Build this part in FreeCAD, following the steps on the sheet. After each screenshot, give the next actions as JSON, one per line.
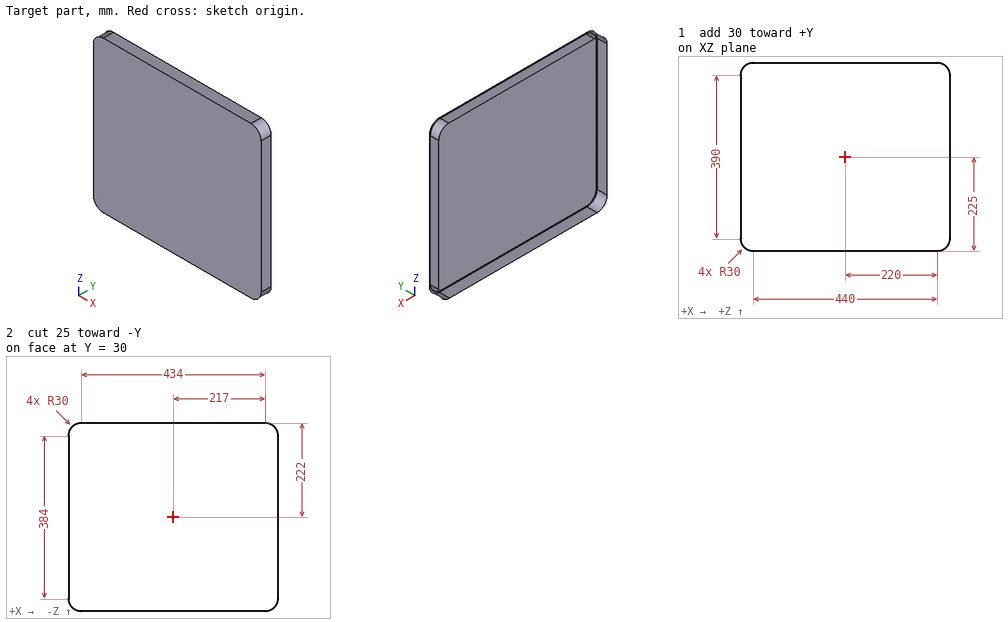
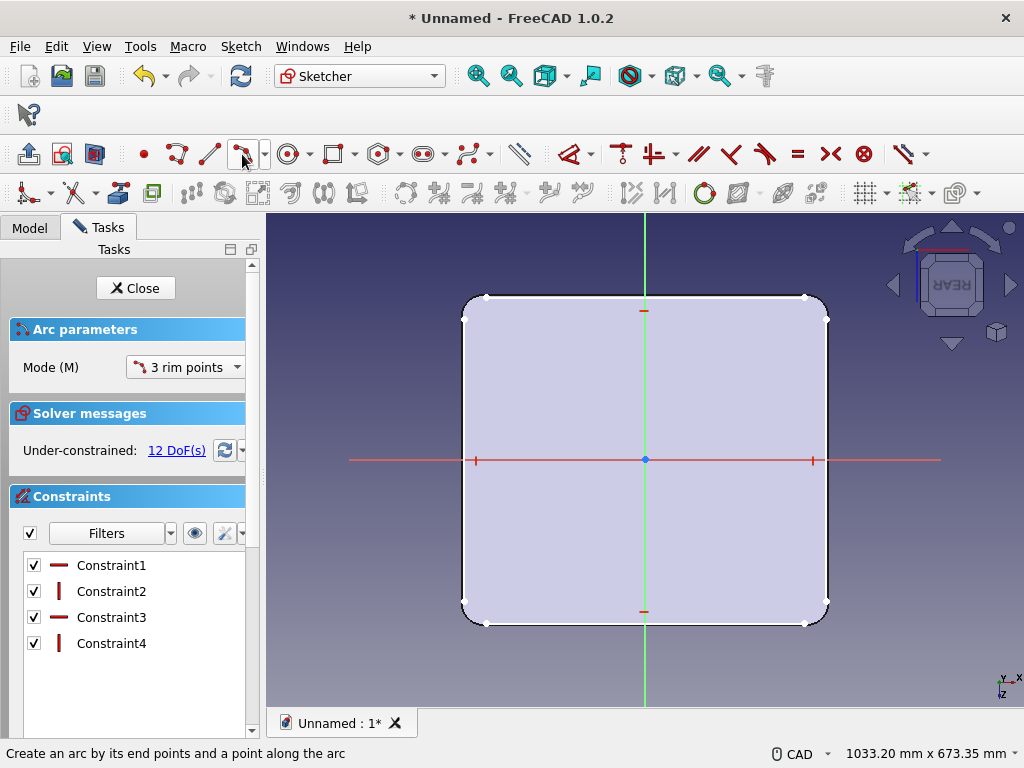
{"action": "left_click", "coordinate": [486, 298]}
{"action": "left_click", "coordinate": [464, 320]}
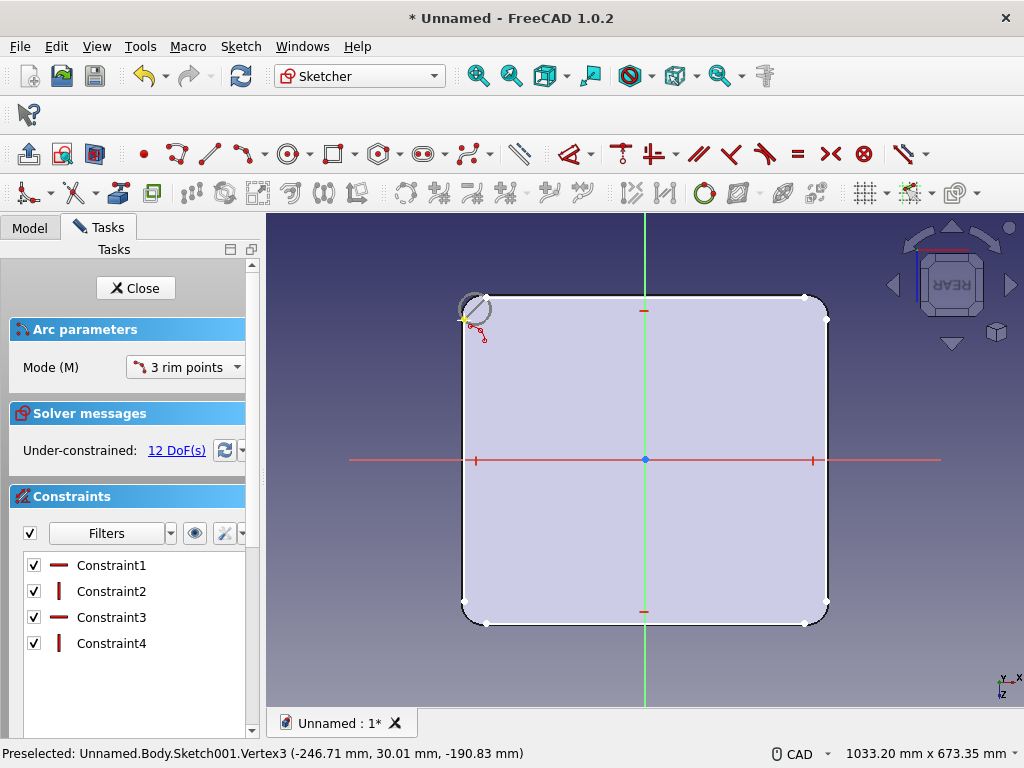
{"action": "scroll", "coordinate": [470, 304], "scroll_direction": "up", "scroll_amount": 5}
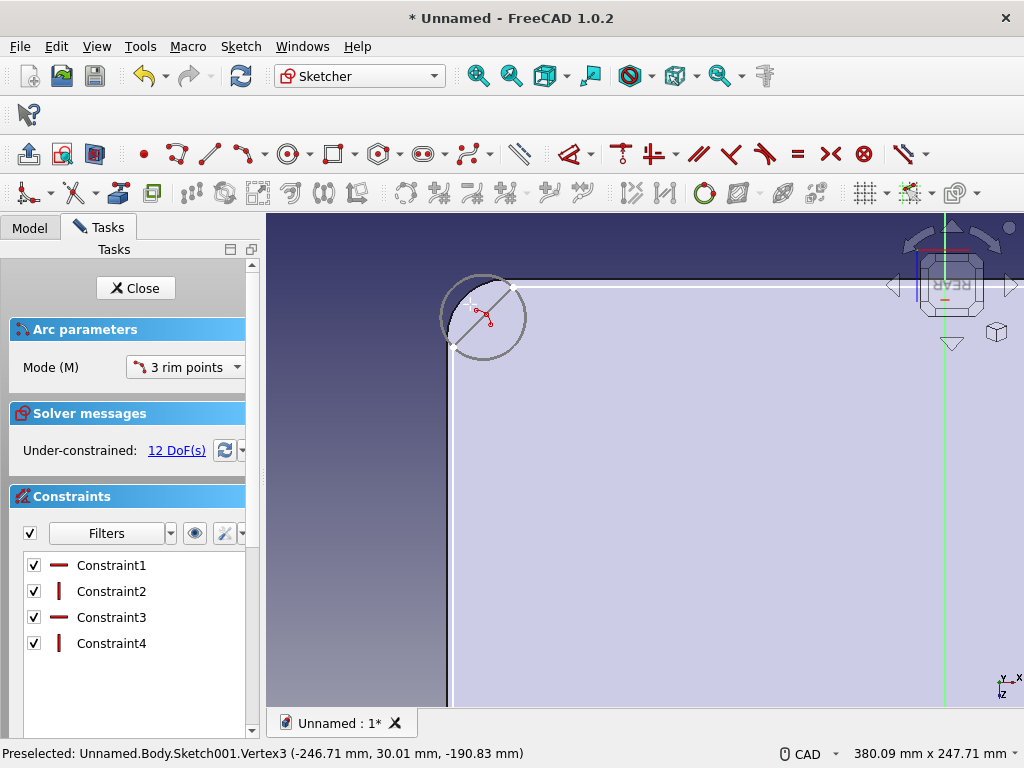
{"action": "left_click", "coordinate": [470, 303]}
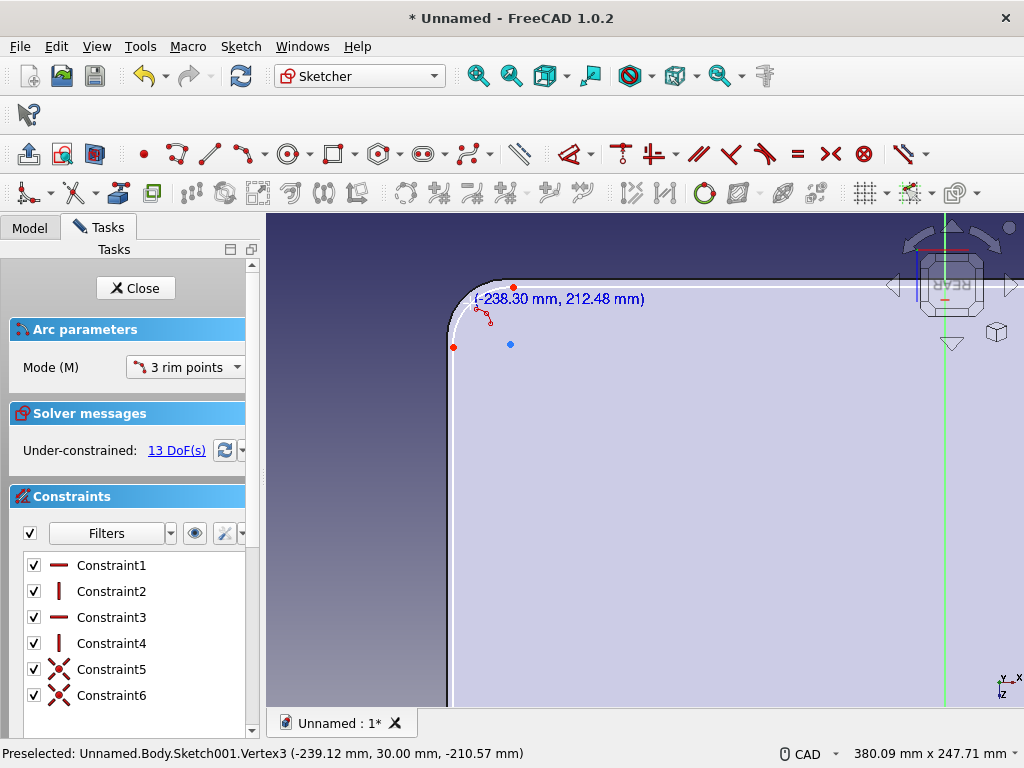
{"action": "scroll", "coordinate": [362, 304], "scroll_direction": "down", "scroll_amount": 5}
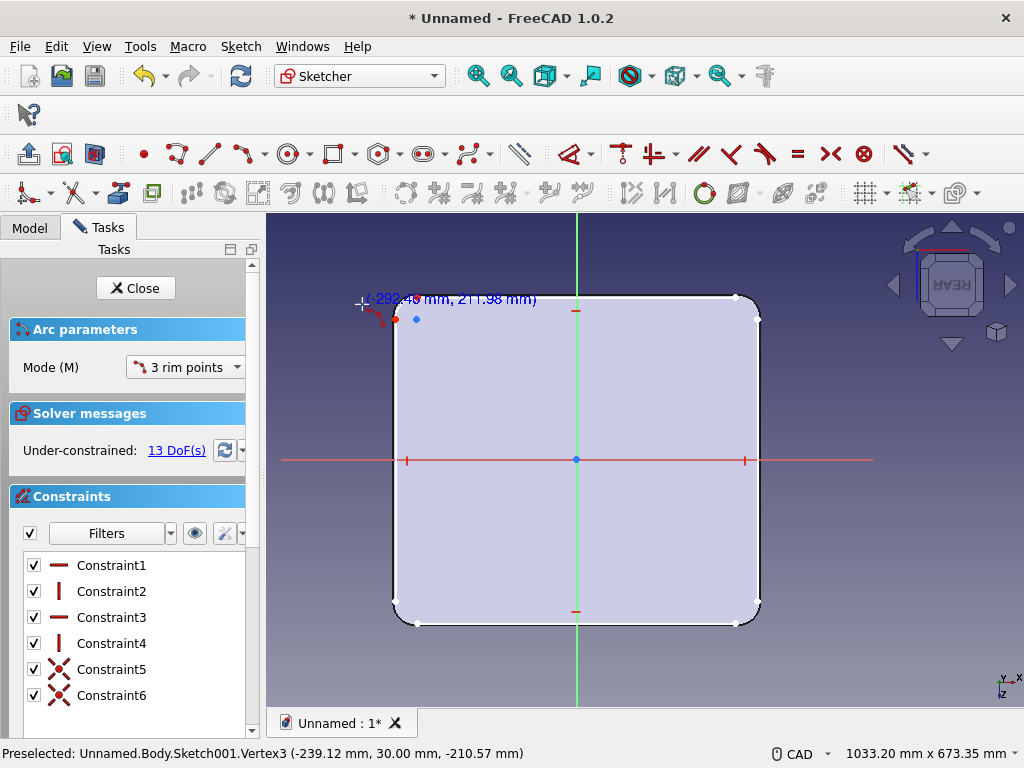
{"action": "left_click", "coordinate": [396, 602]}
{"action": "left_click", "coordinate": [418, 624]}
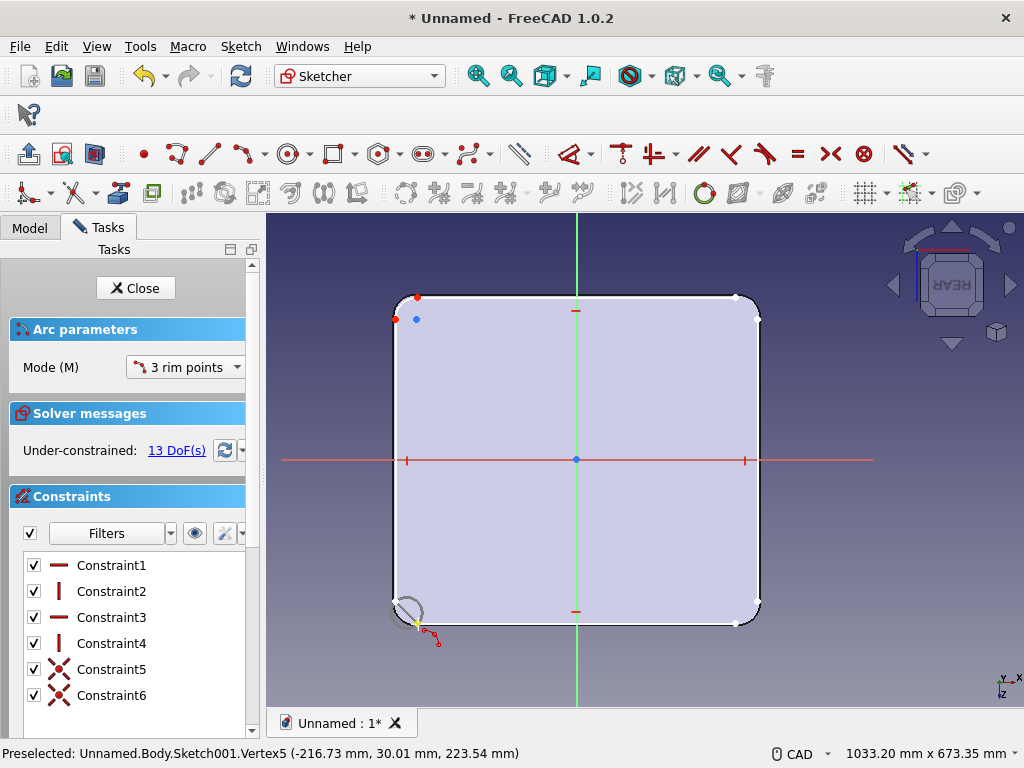
{"action": "scroll", "coordinate": [402, 616], "scroll_direction": "up", "scroll_amount": 5}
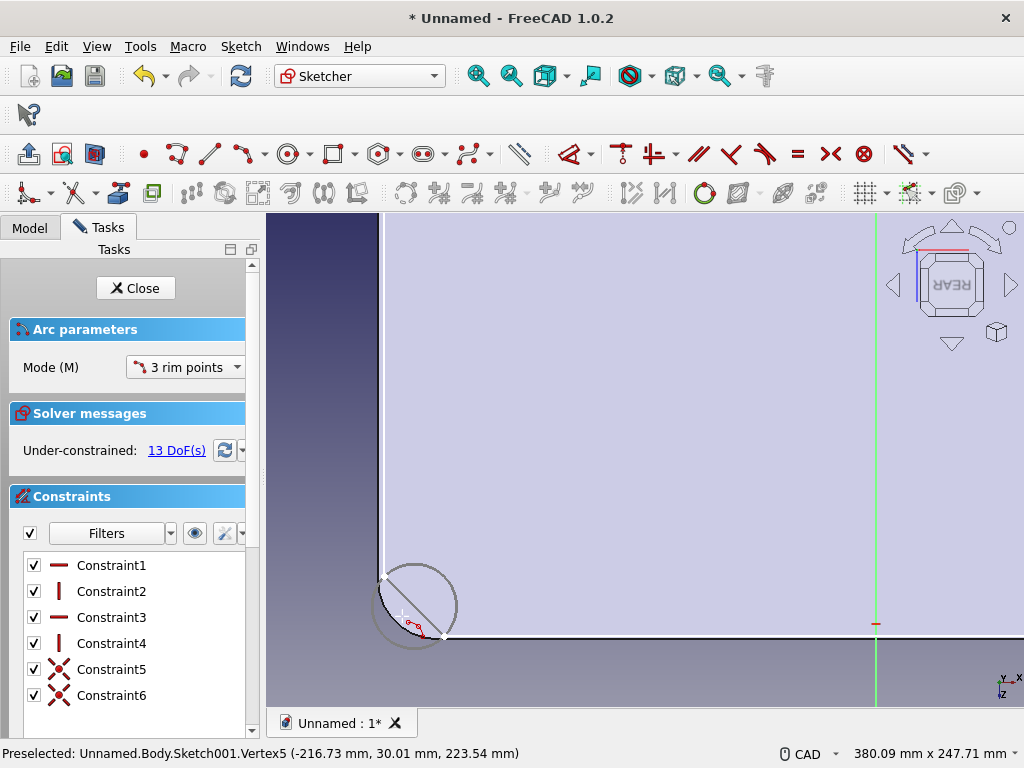
{"action": "left_click", "coordinate": [401, 616]}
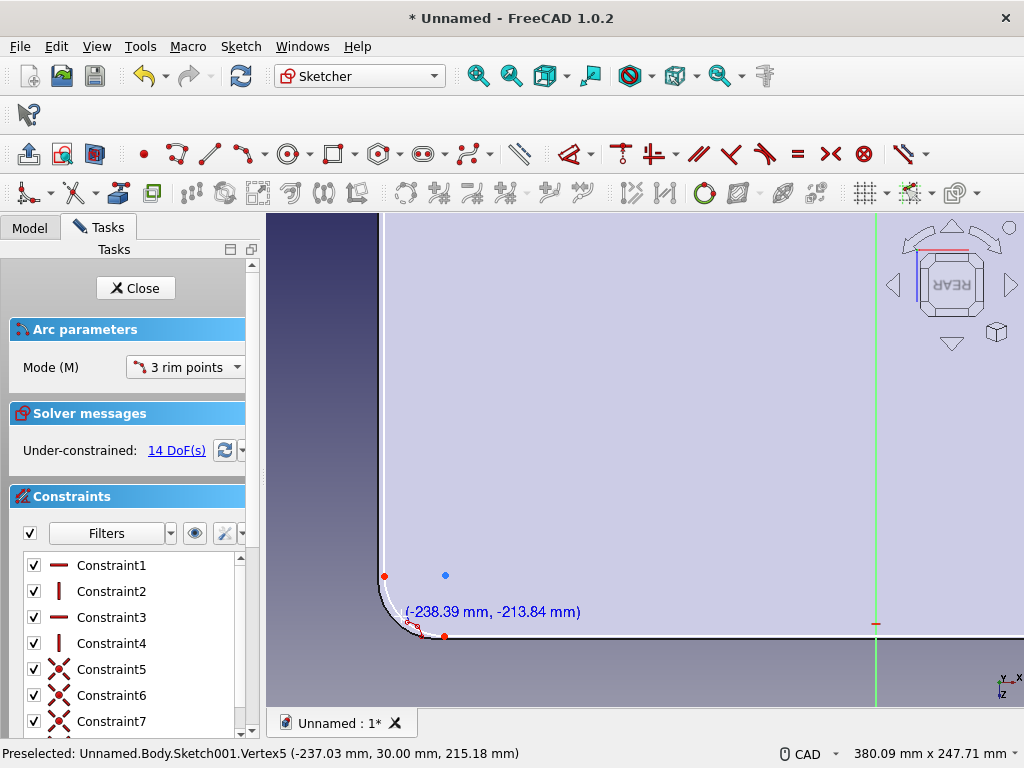
{"action": "scroll", "coordinate": [402, 617], "scroll_direction": "down", "scroll_amount": 5}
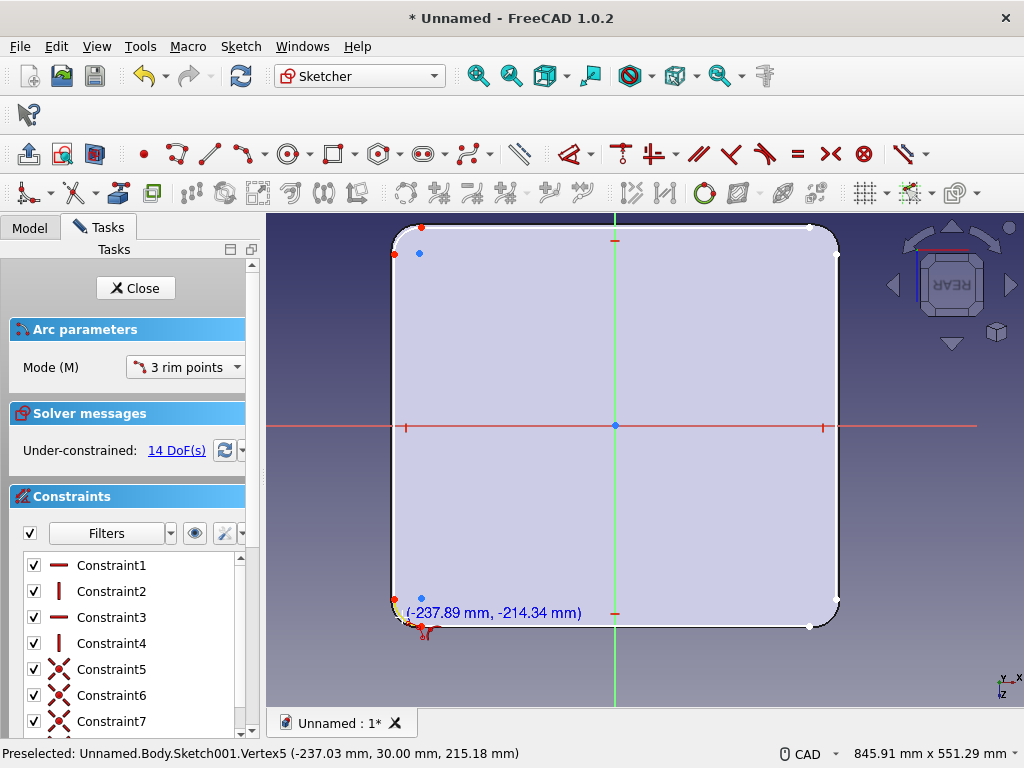
{"action": "left_click", "coordinate": [736, 625]}
{"action": "left_click", "coordinate": [758, 603]}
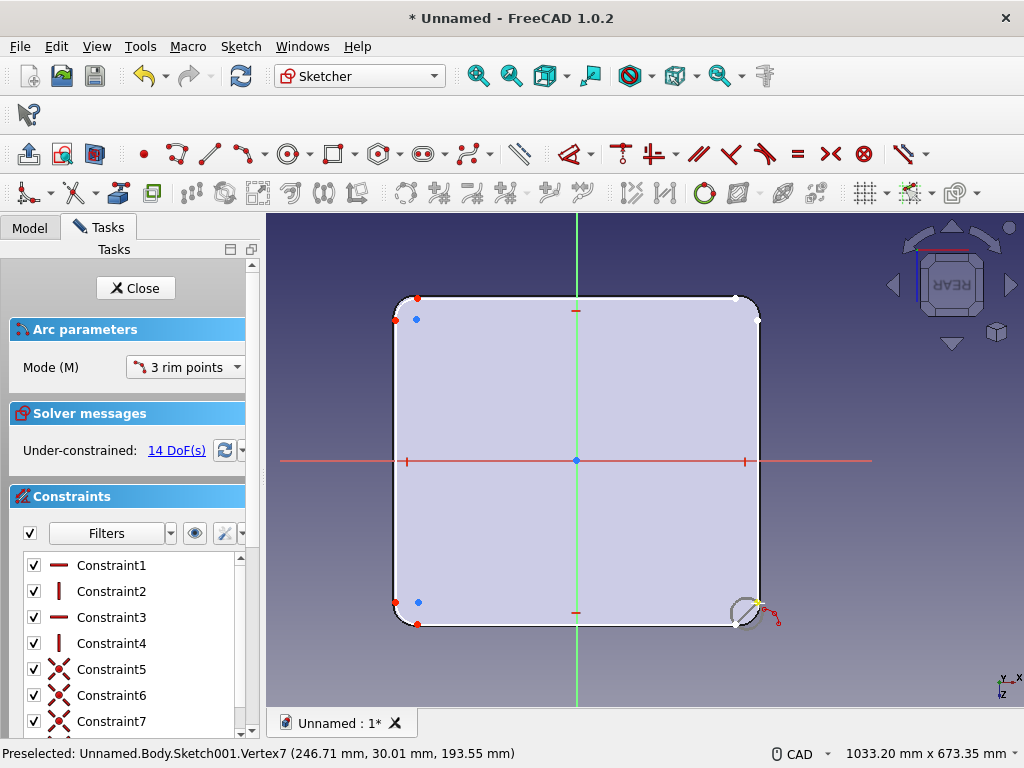
{"action": "scroll", "coordinate": [751, 617], "scroll_direction": "up", "scroll_amount": 5}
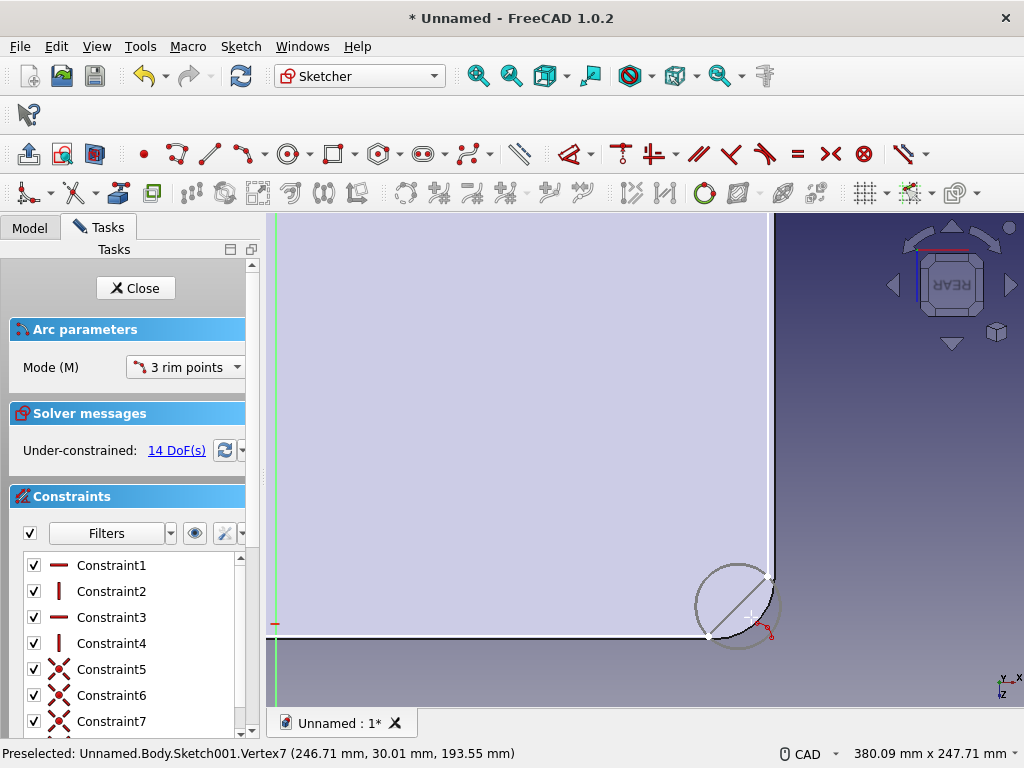
{"action": "left_click", "coordinate": [751, 616]}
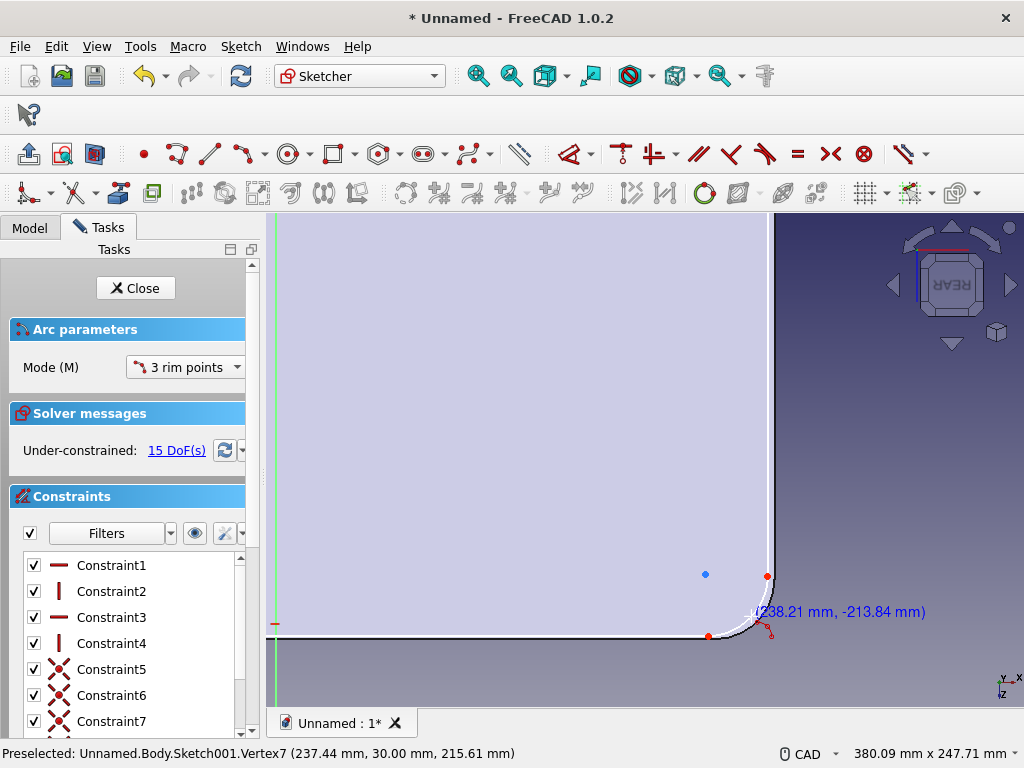
{"action": "scroll", "coordinate": [751, 617], "scroll_direction": "down", "scroll_amount": 5}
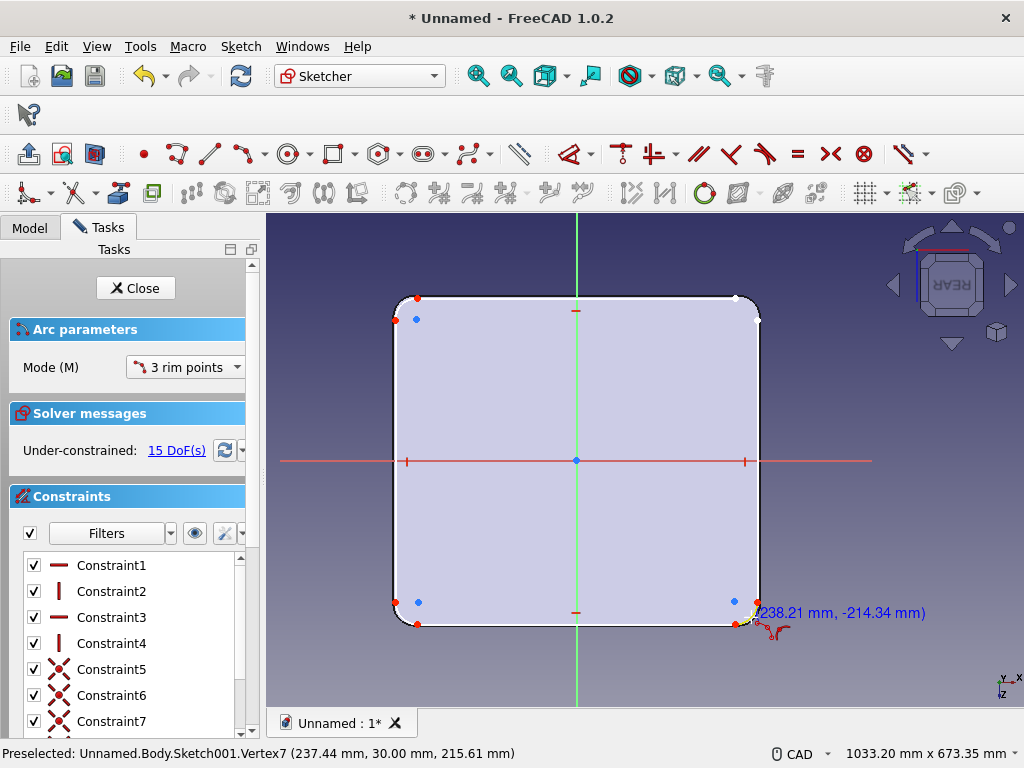
{"action": "left_click", "coordinate": [758, 321]}
{"action": "left_click", "coordinate": [736, 299]}